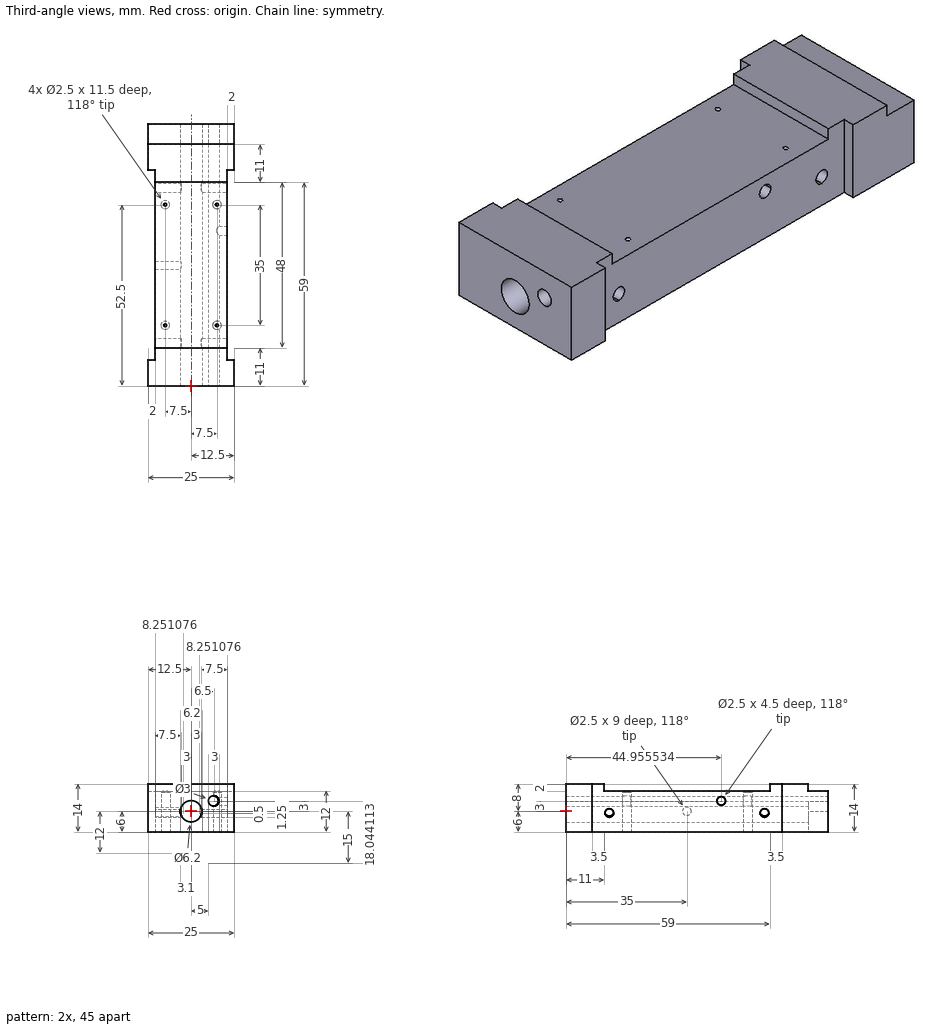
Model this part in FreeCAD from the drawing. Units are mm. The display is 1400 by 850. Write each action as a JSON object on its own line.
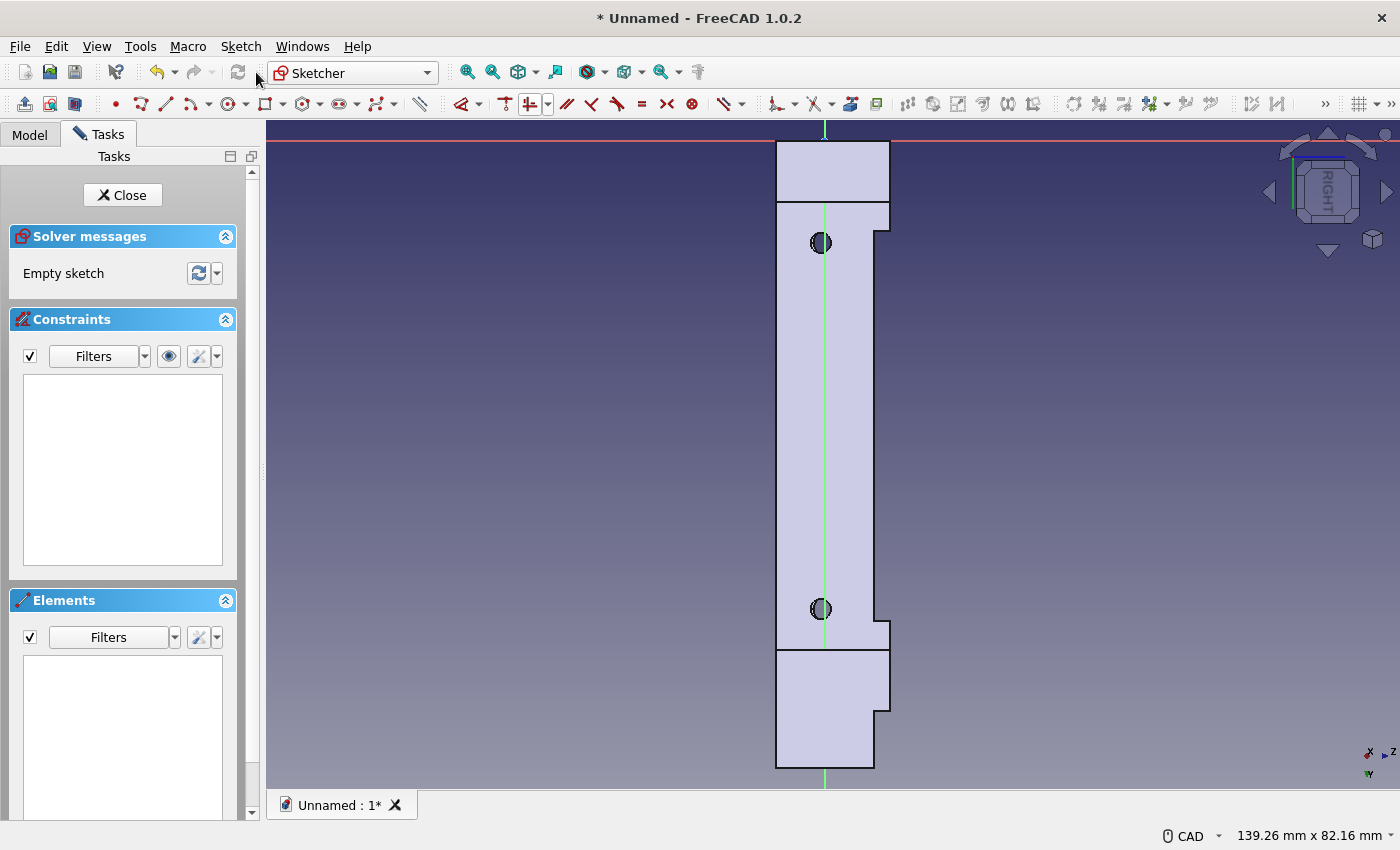
{"action": "scroll", "coordinate": [854, 510], "scroll_direction": "up", "scroll_amount": 15}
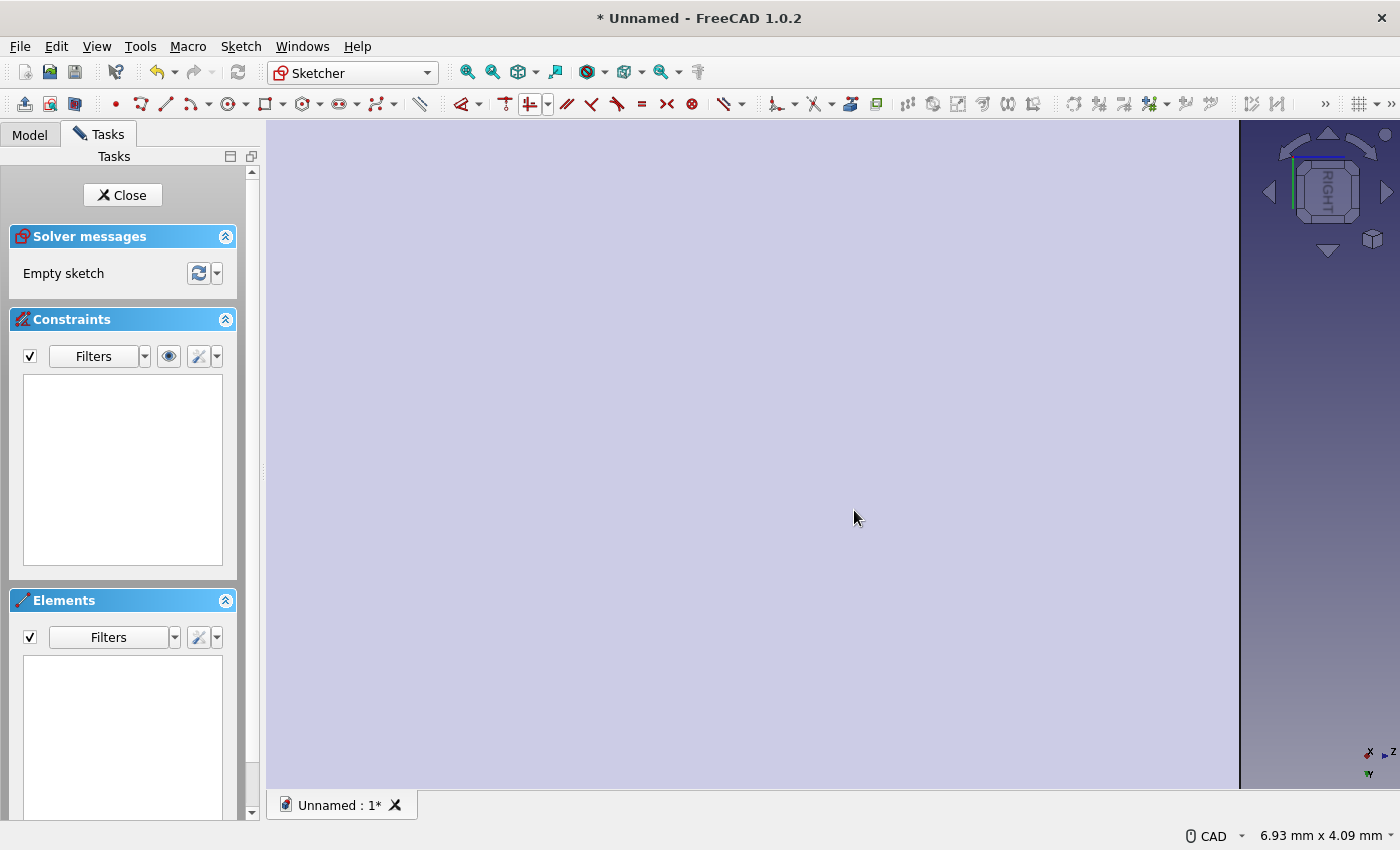
{"action": "left_click", "coordinate": [228, 104]}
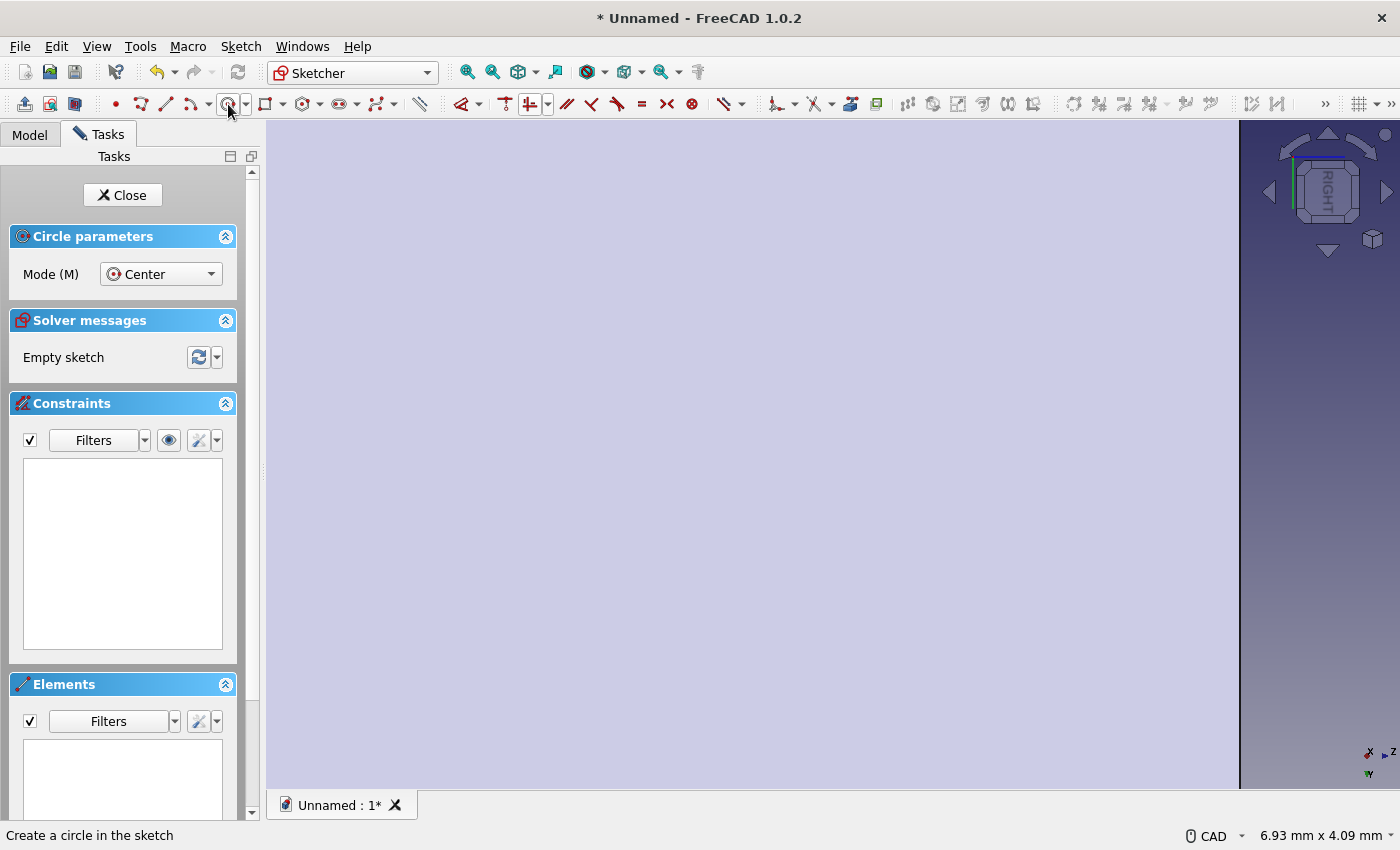
{"action": "left_click", "coordinate": [749, 440]}
{"action": "left_click", "coordinate": [894, 295]}
{"action": "key", "text": "Escape"}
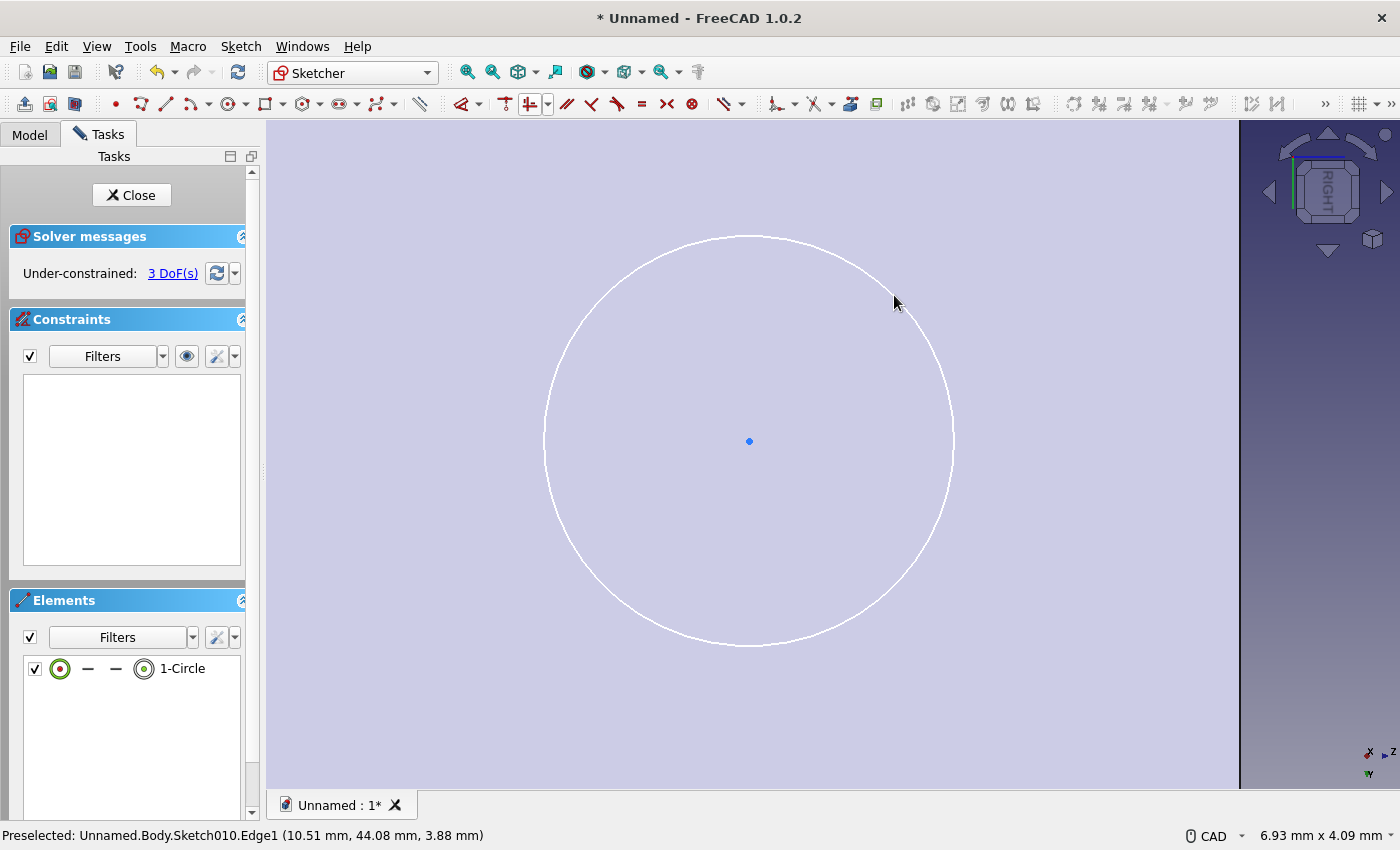
{"action": "left_click", "coordinate": [460, 104]}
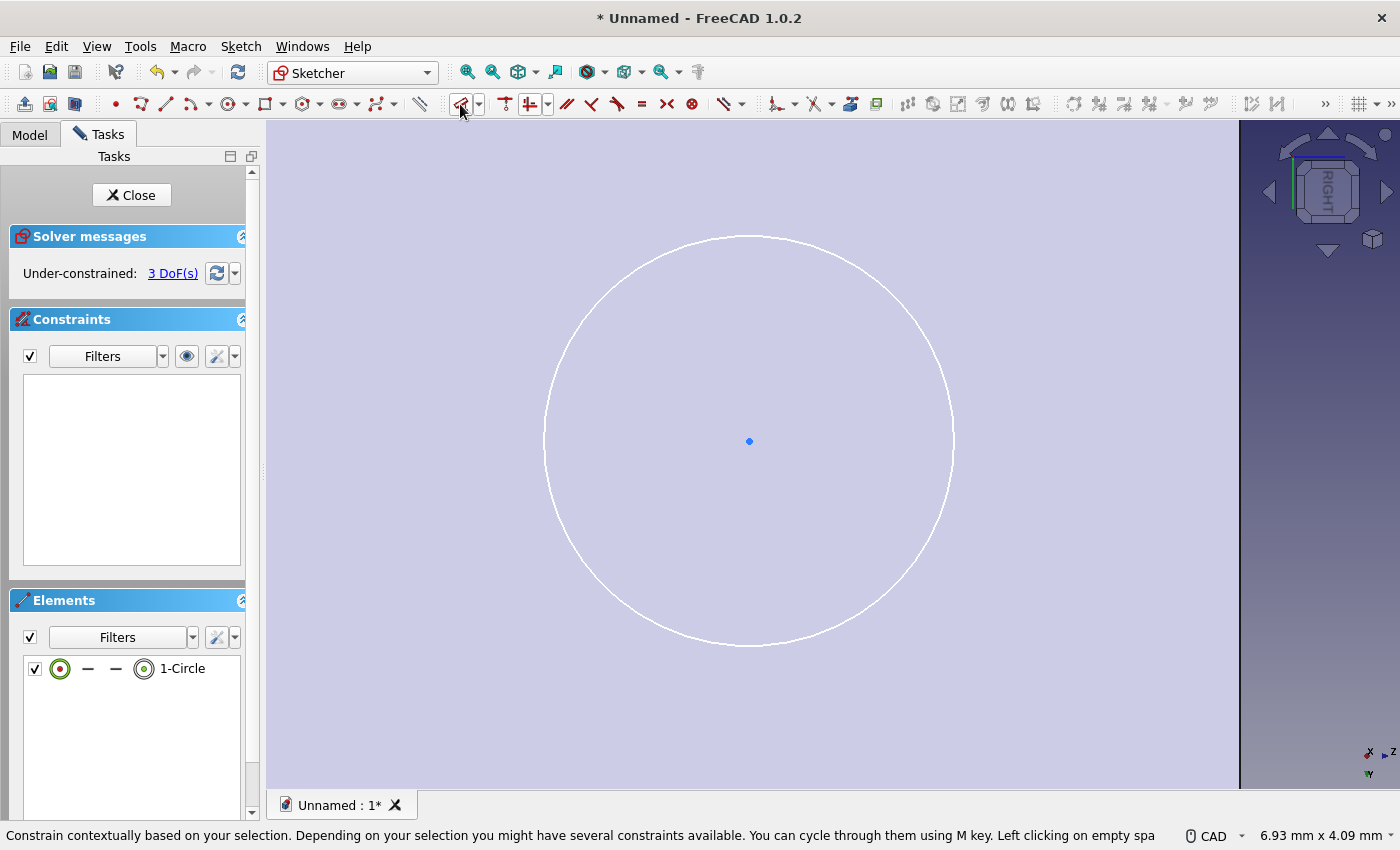
{"action": "left_click", "coordinate": [894, 296]}
{"action": "left_click", "coordinate": [917, 273]}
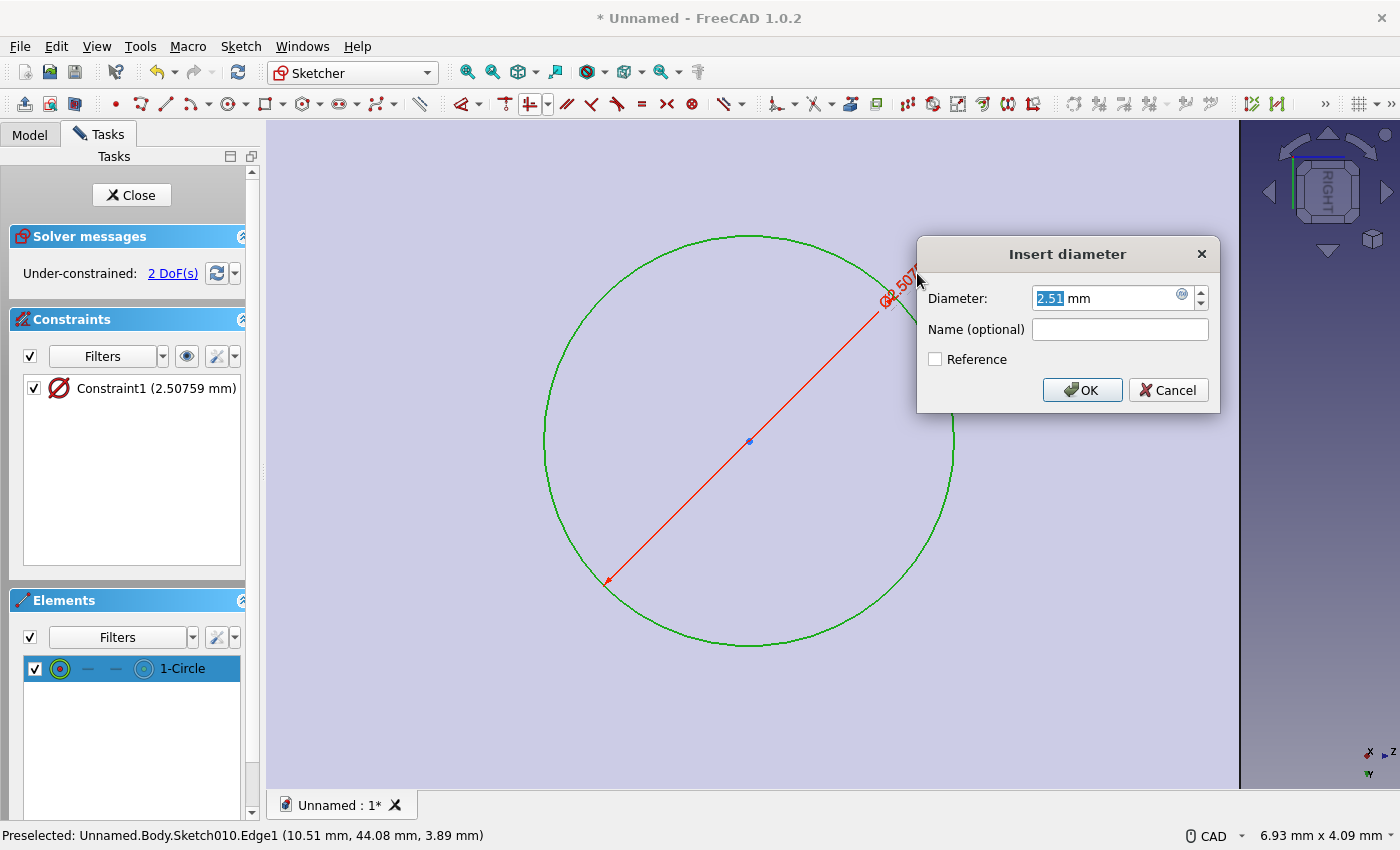
{"action": "type", "text": "2.5"}
{"action": "key", "text": "Return"}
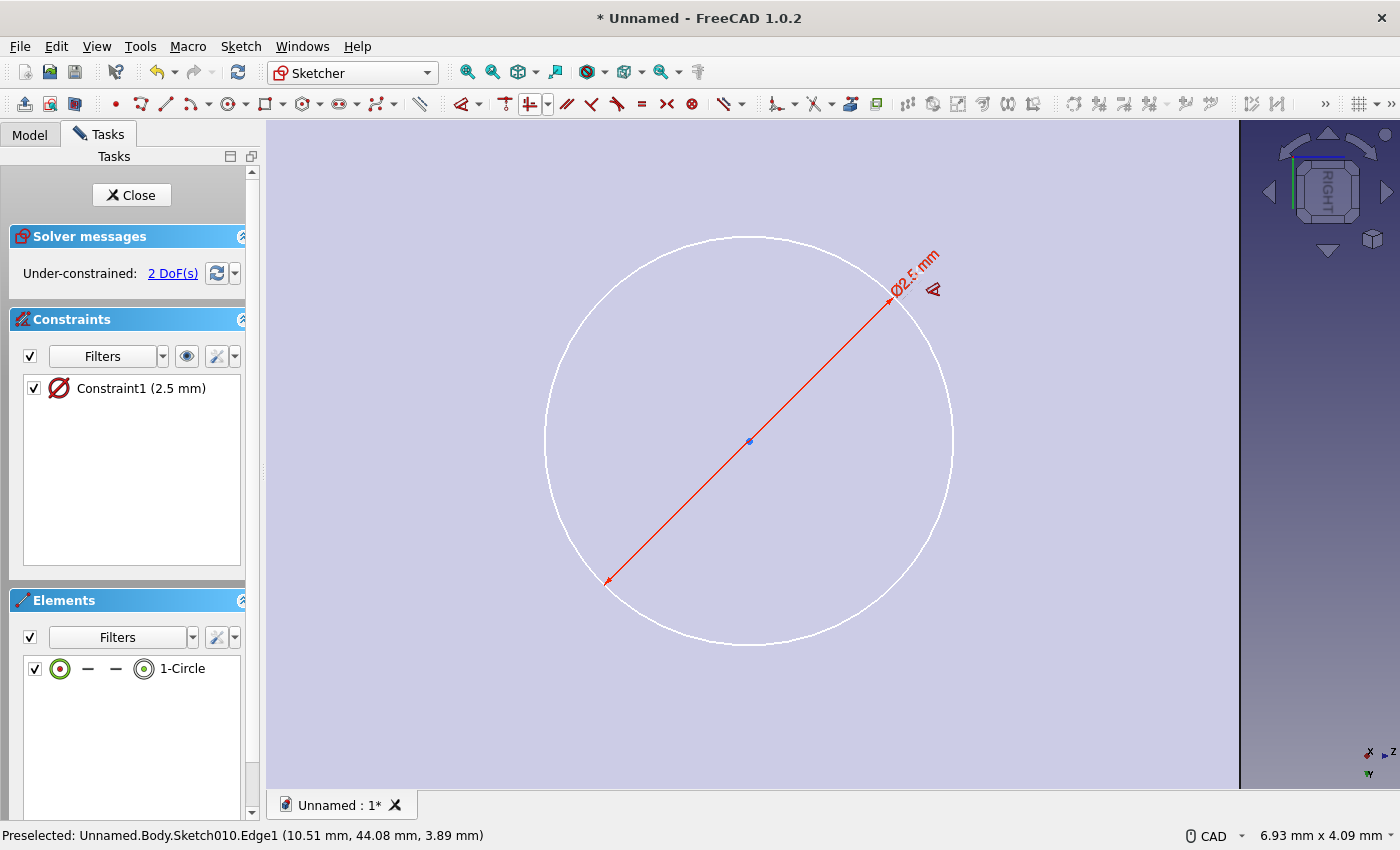
{"action": "left_click", "coordinate": [749, 441]}
{"action": "left_click", "coordinate": [521, 475]}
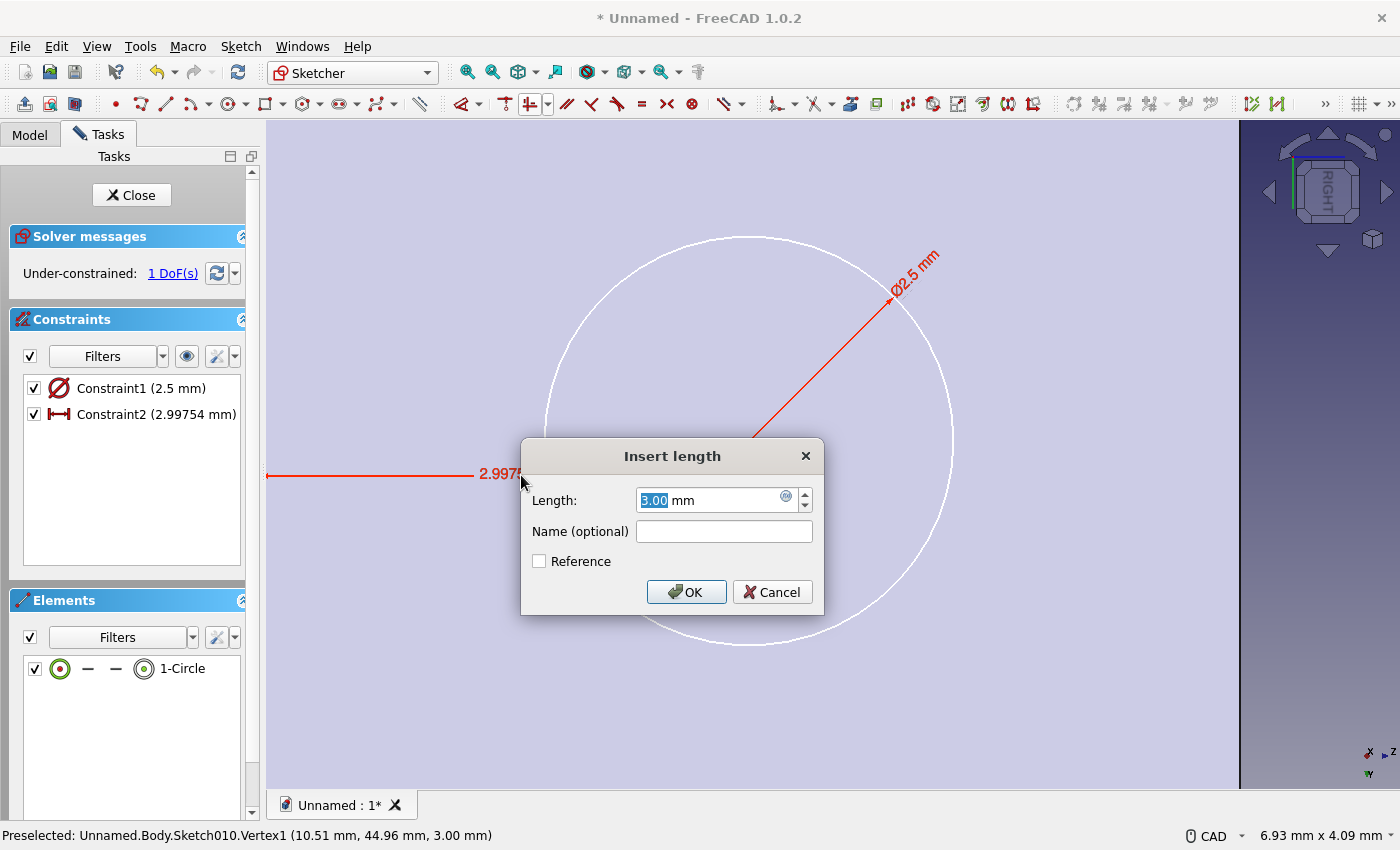
{"action": "type", "text": "3"}
{"action": "key", "text": "Return"}